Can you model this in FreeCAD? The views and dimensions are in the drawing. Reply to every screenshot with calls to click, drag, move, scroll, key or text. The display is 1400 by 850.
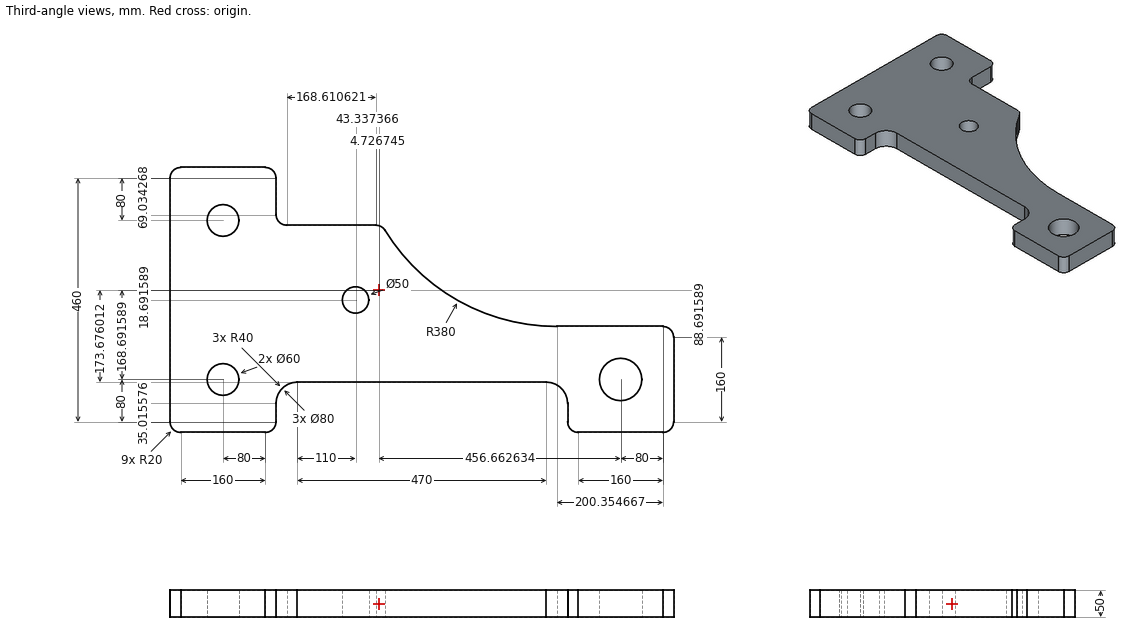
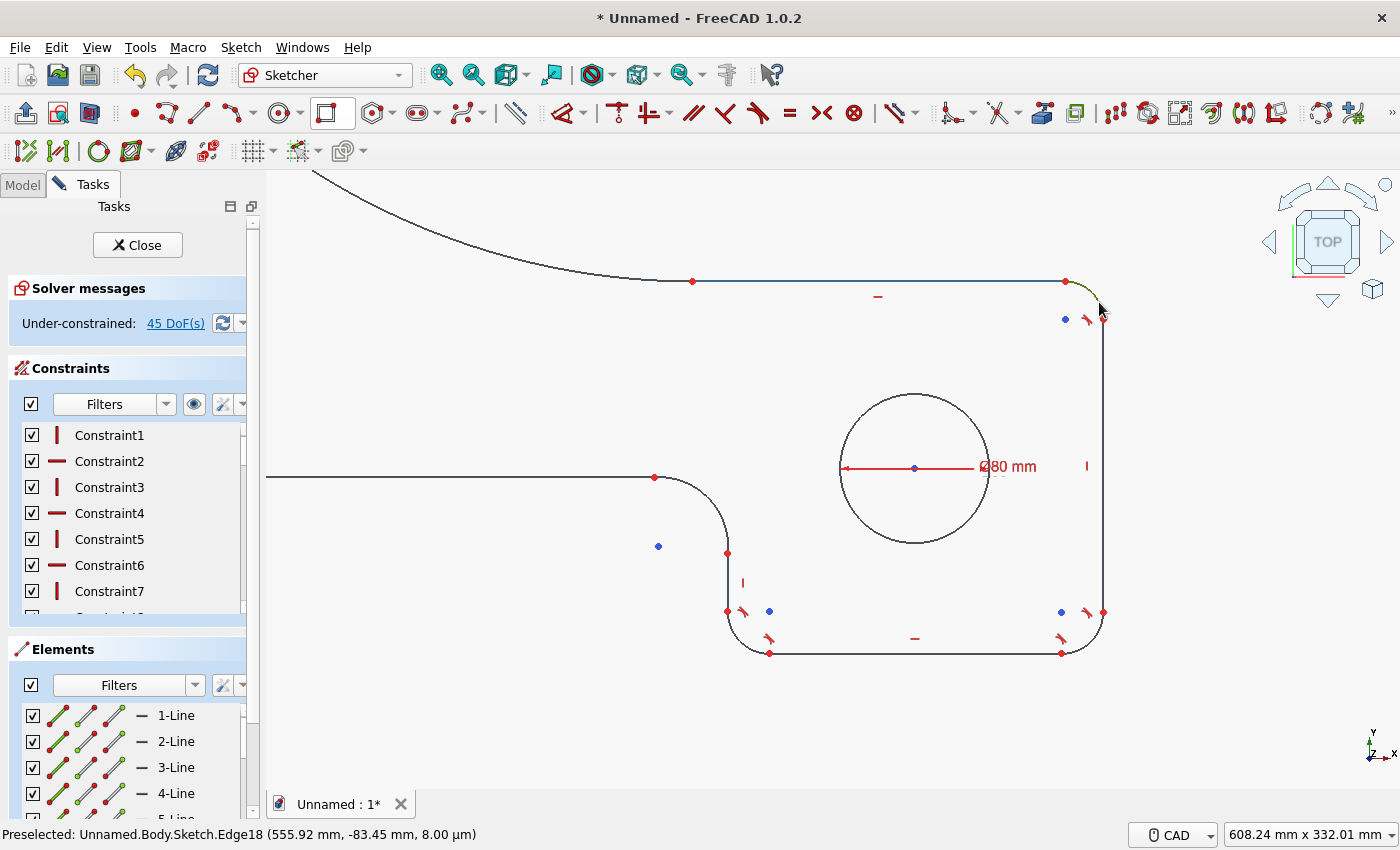
click(758, 114)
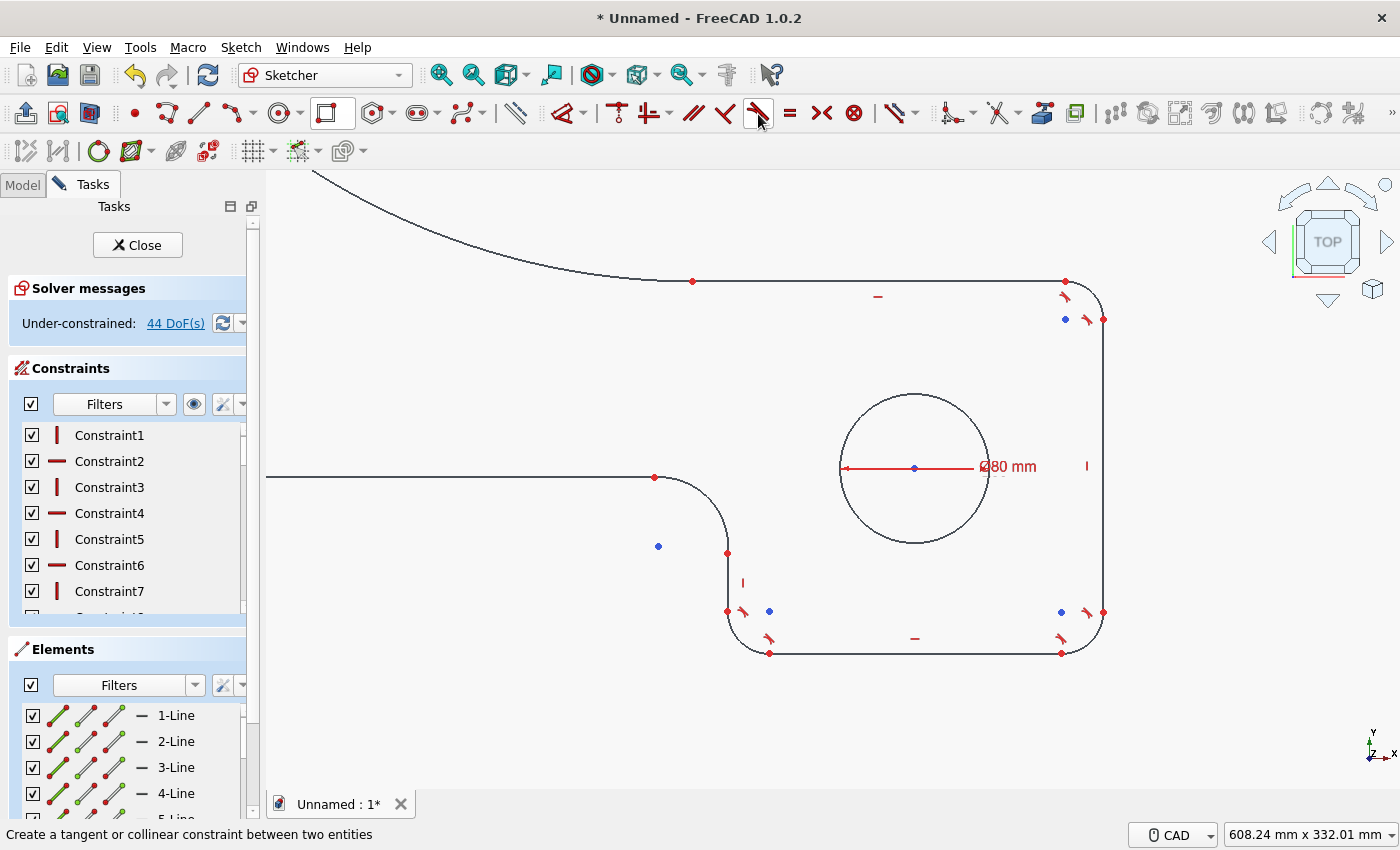
scroll(1083, 650, down, 5)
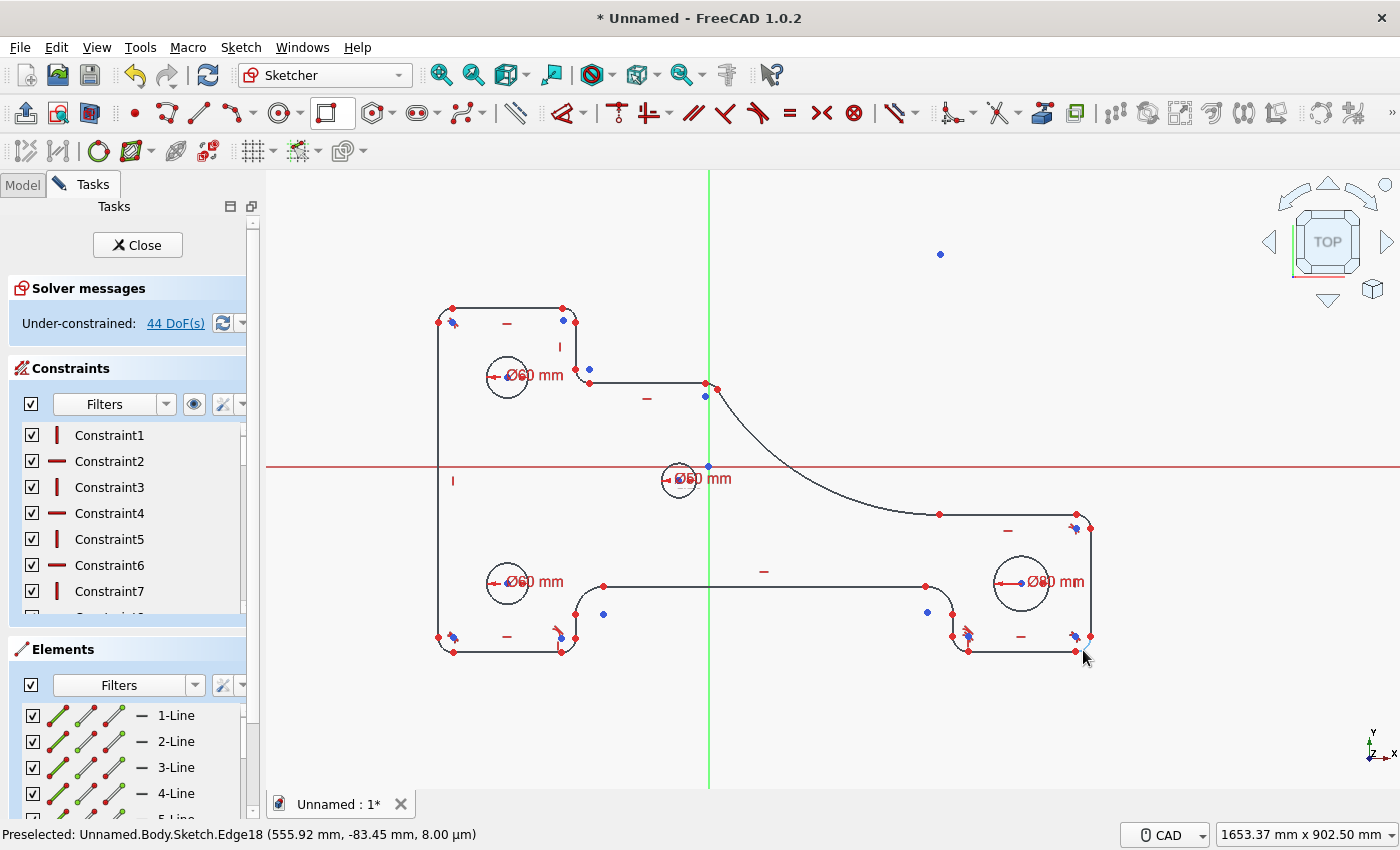
click(671, 383)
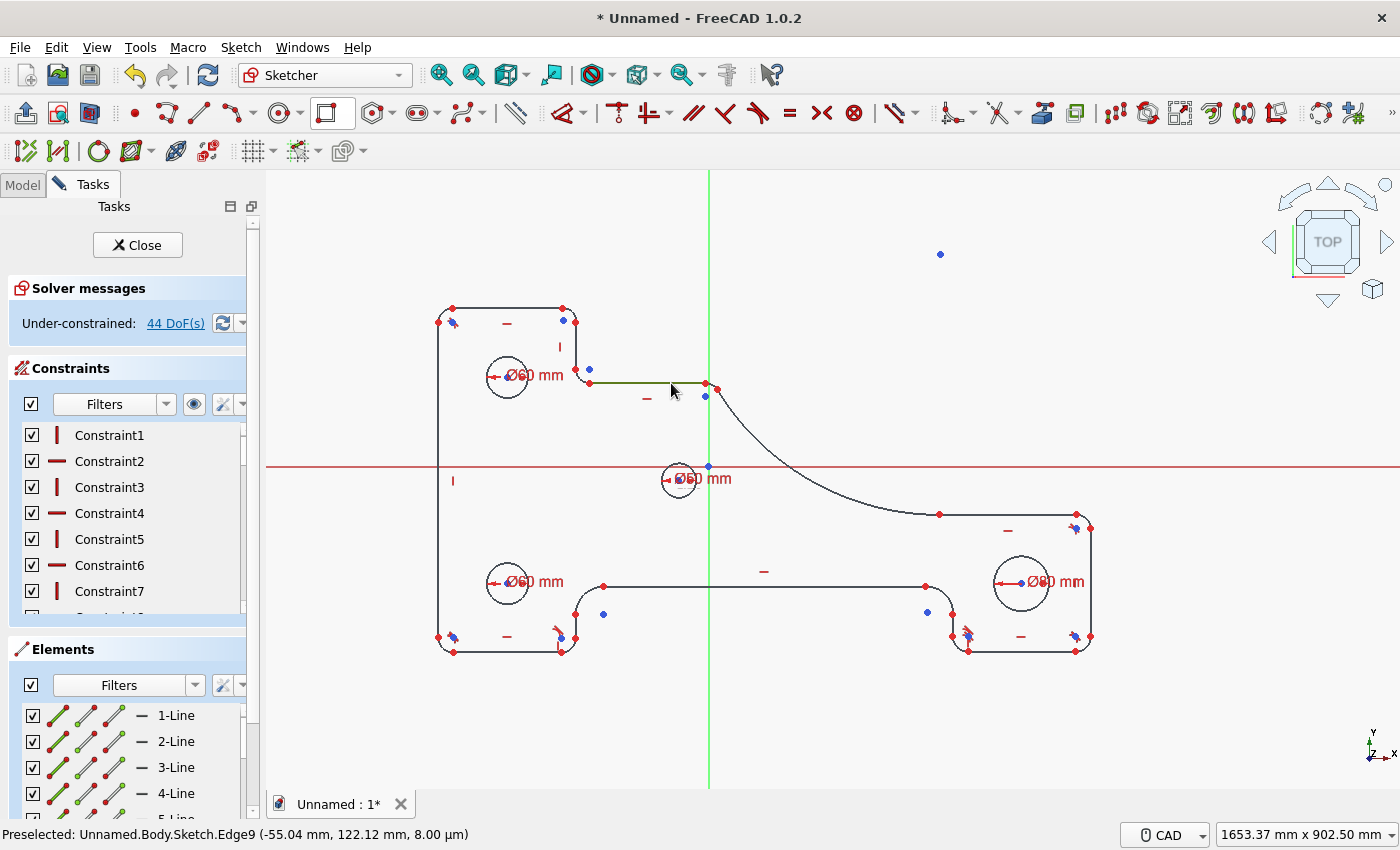
scroll(712, 385, up, 4)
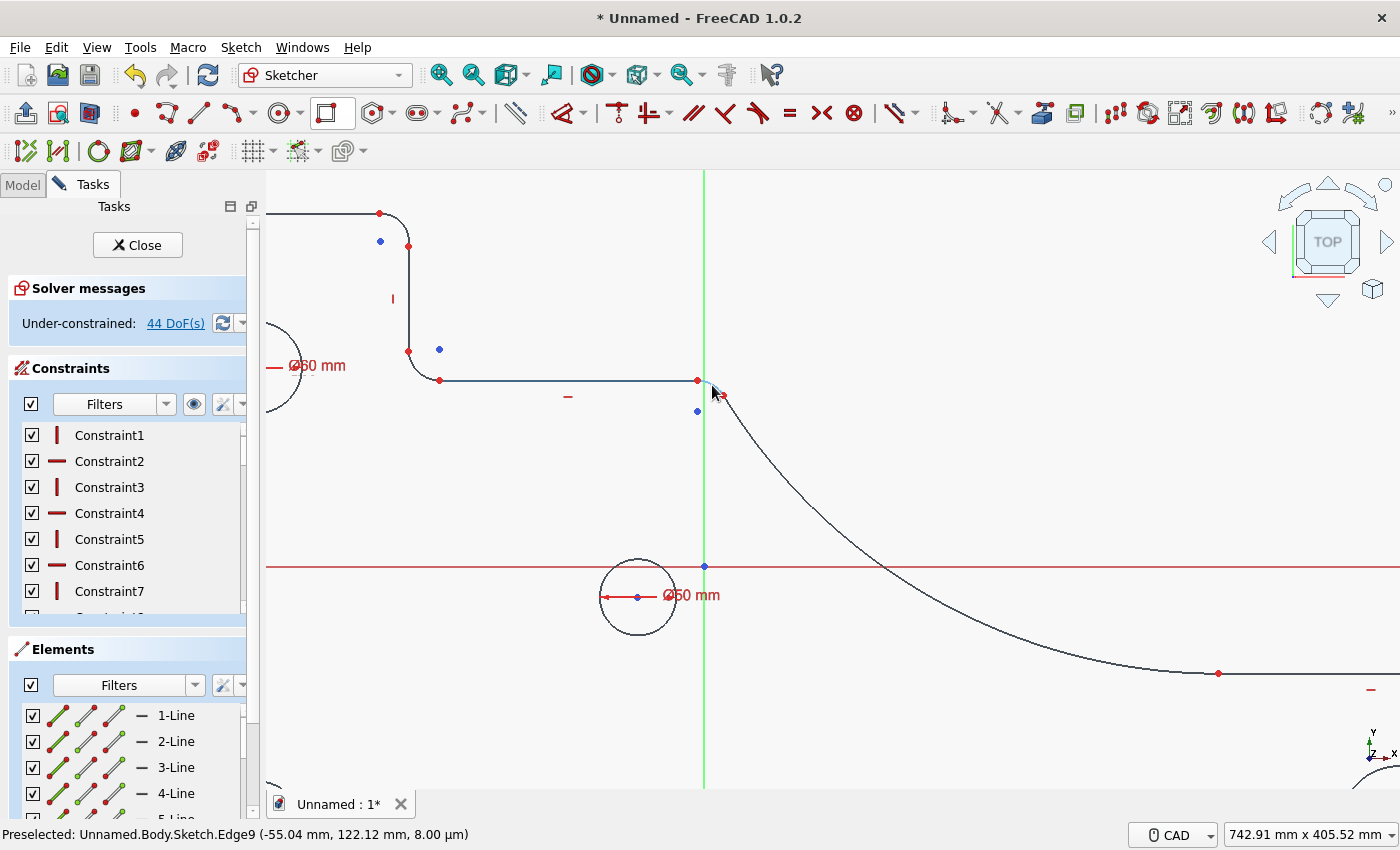
click(712, 385)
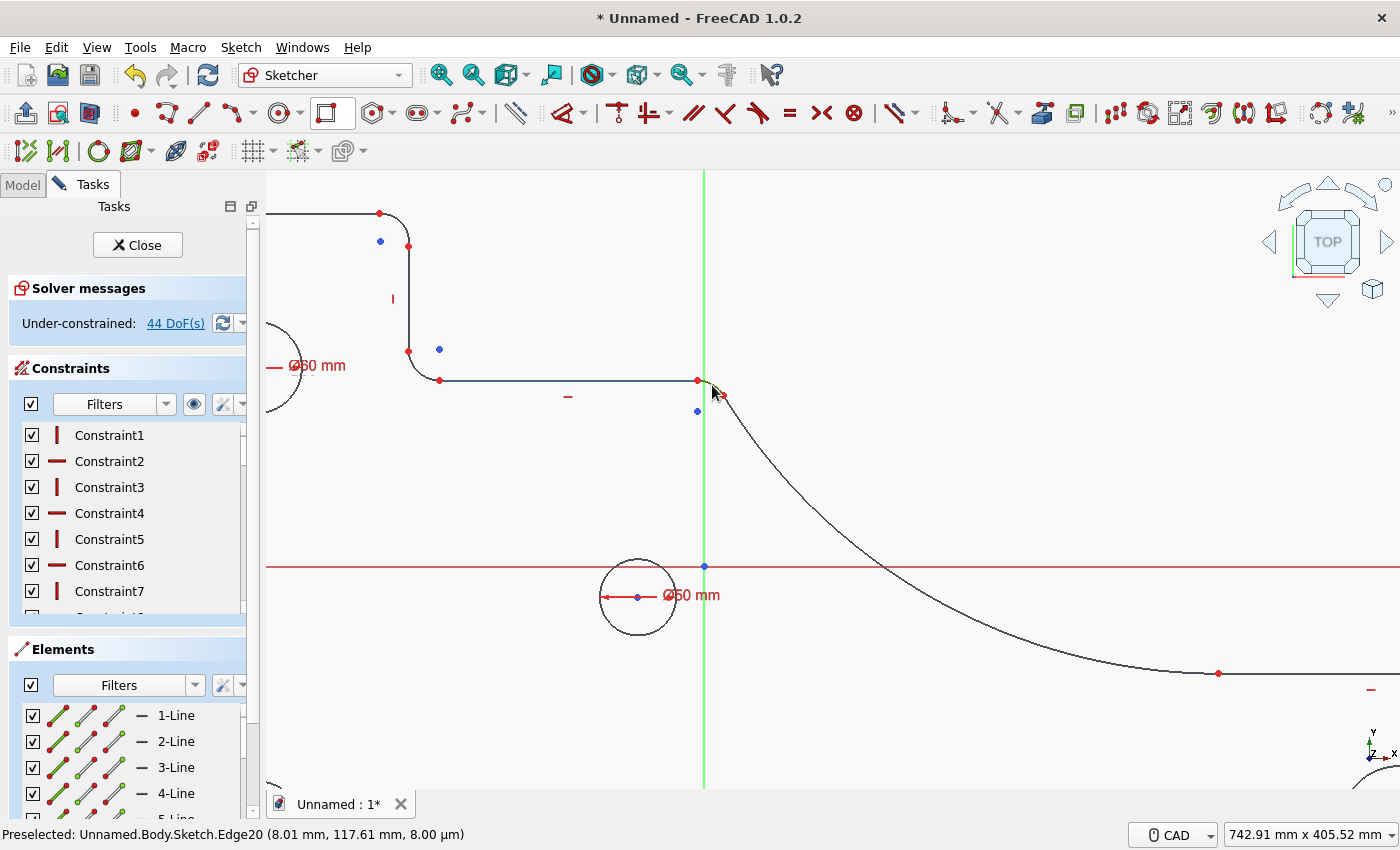
click(758, 114)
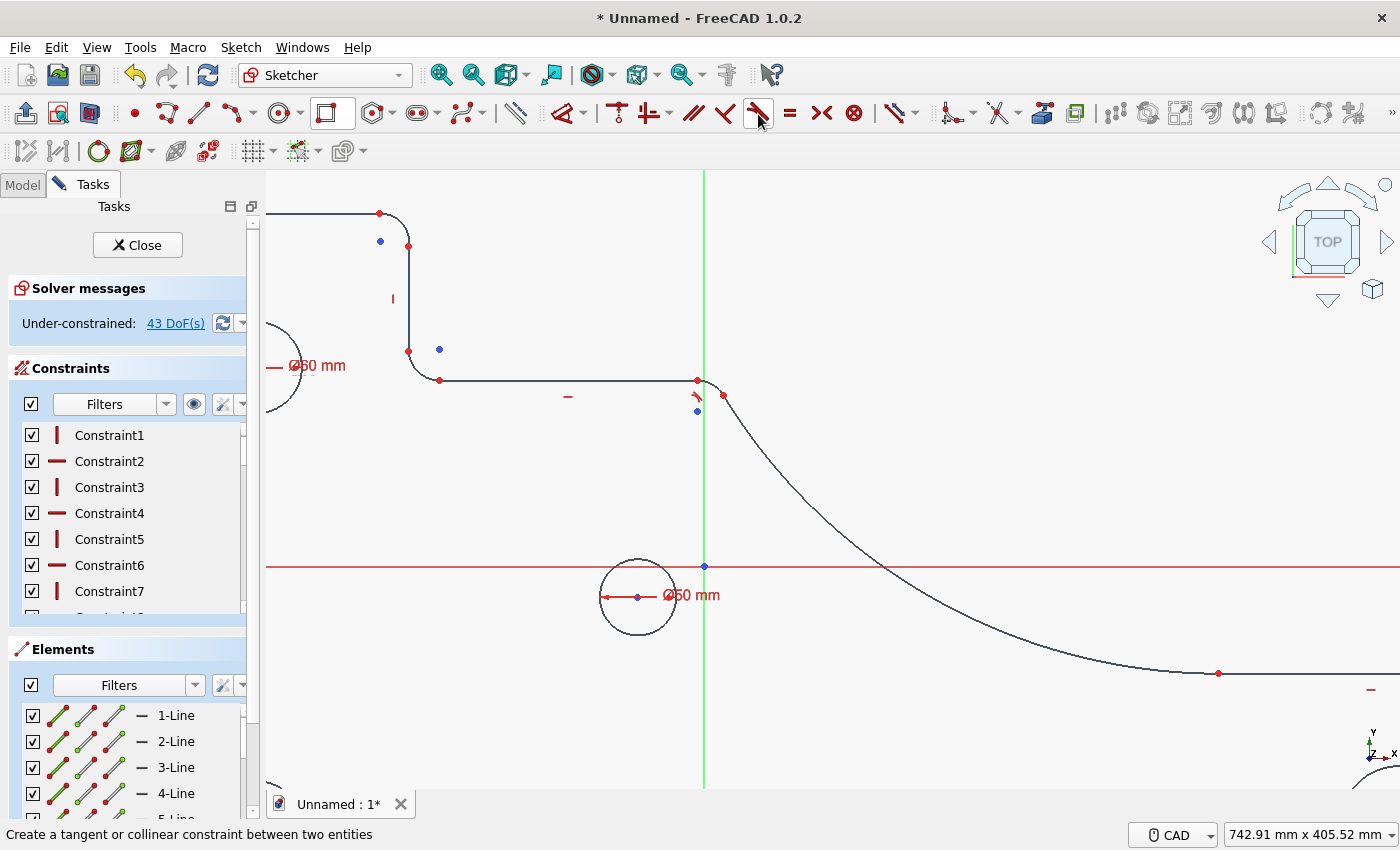
click(620, 381)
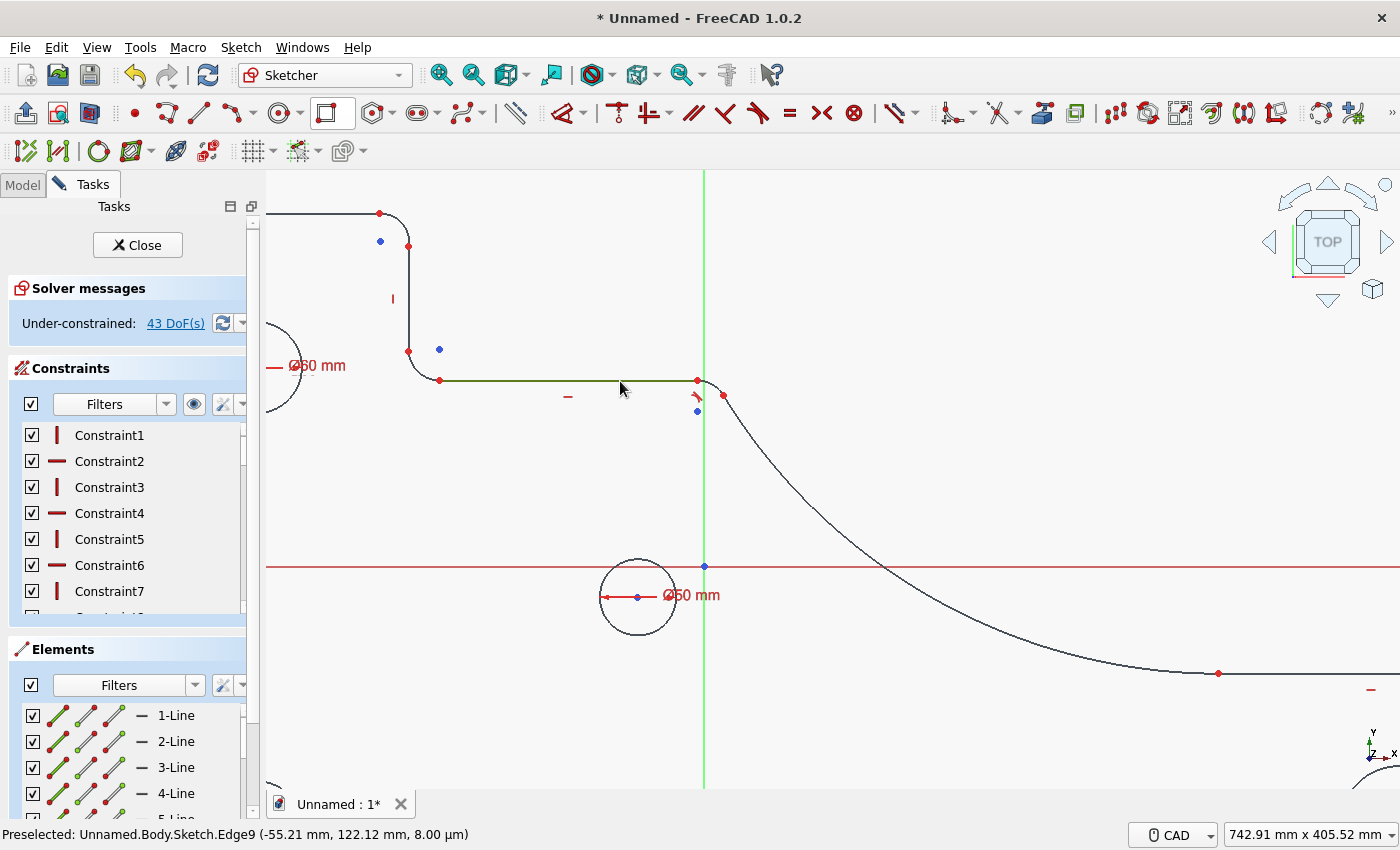
click(413, 365)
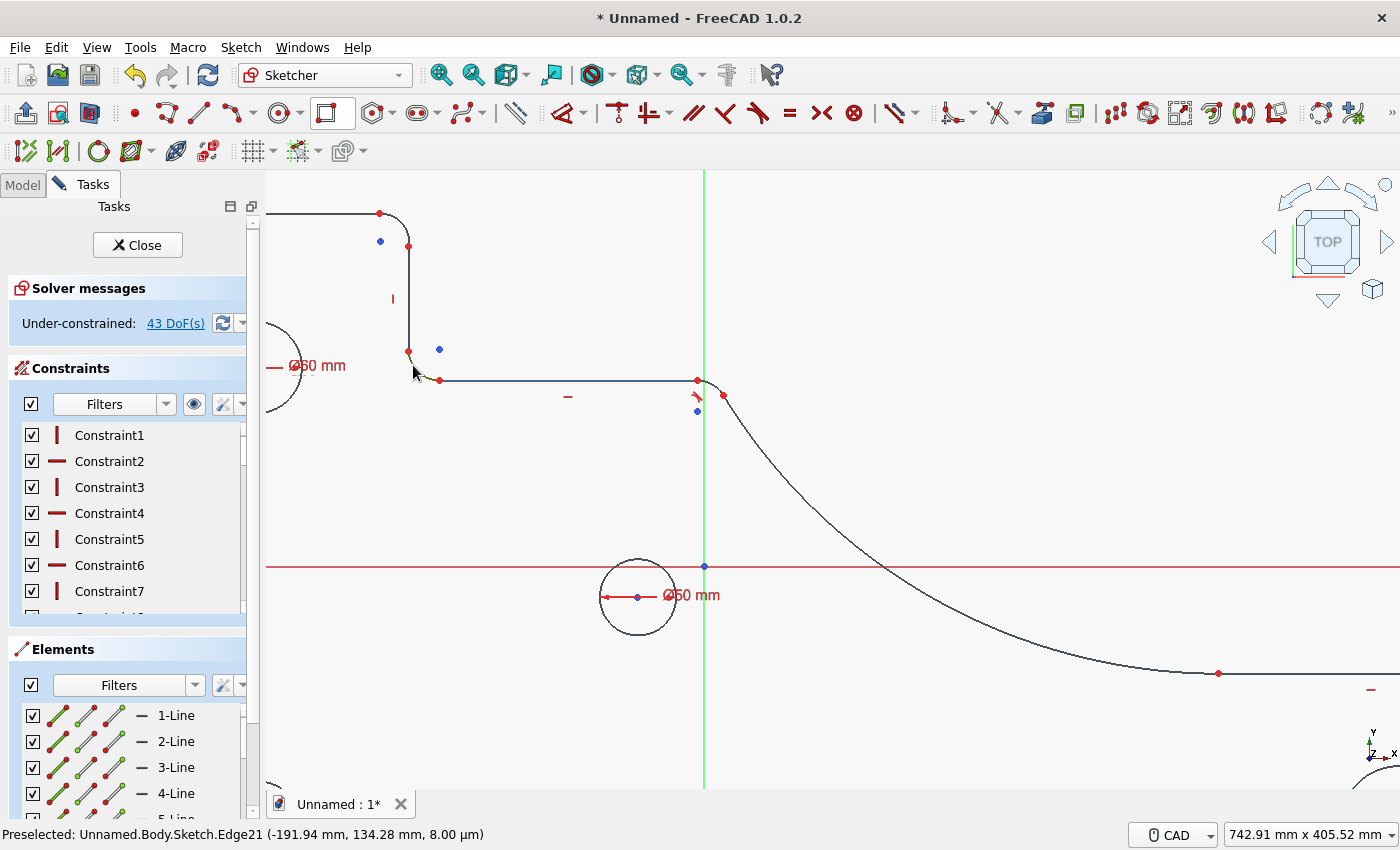
click(758, 114)